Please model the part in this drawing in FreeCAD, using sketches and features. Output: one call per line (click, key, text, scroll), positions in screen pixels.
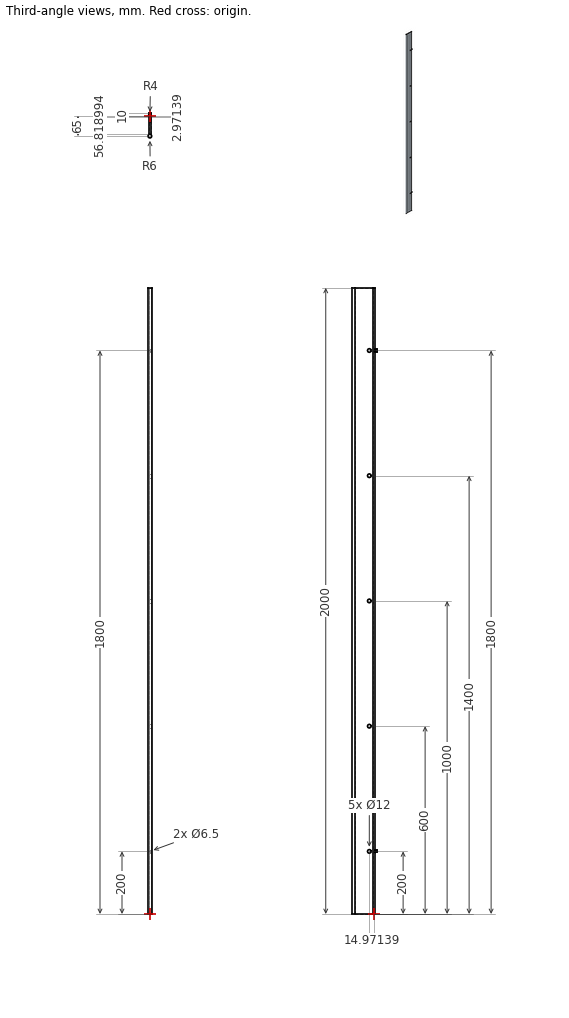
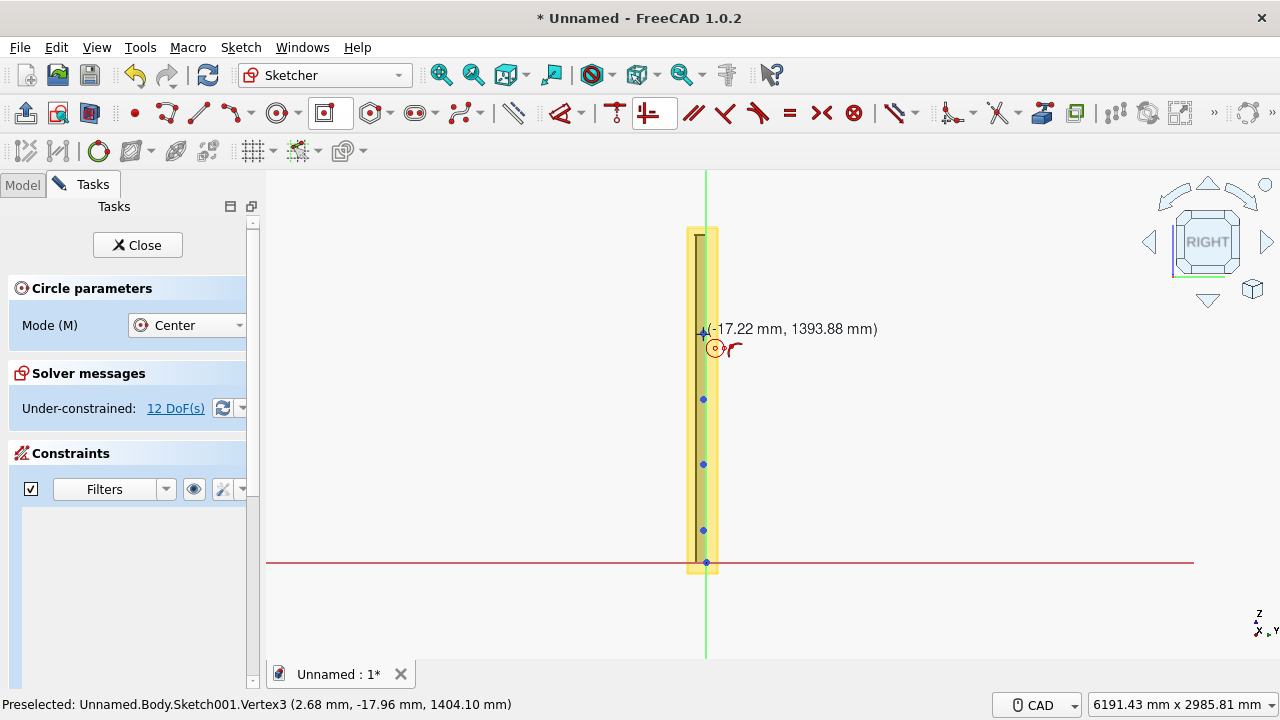
scroll(704, 268, up, 16)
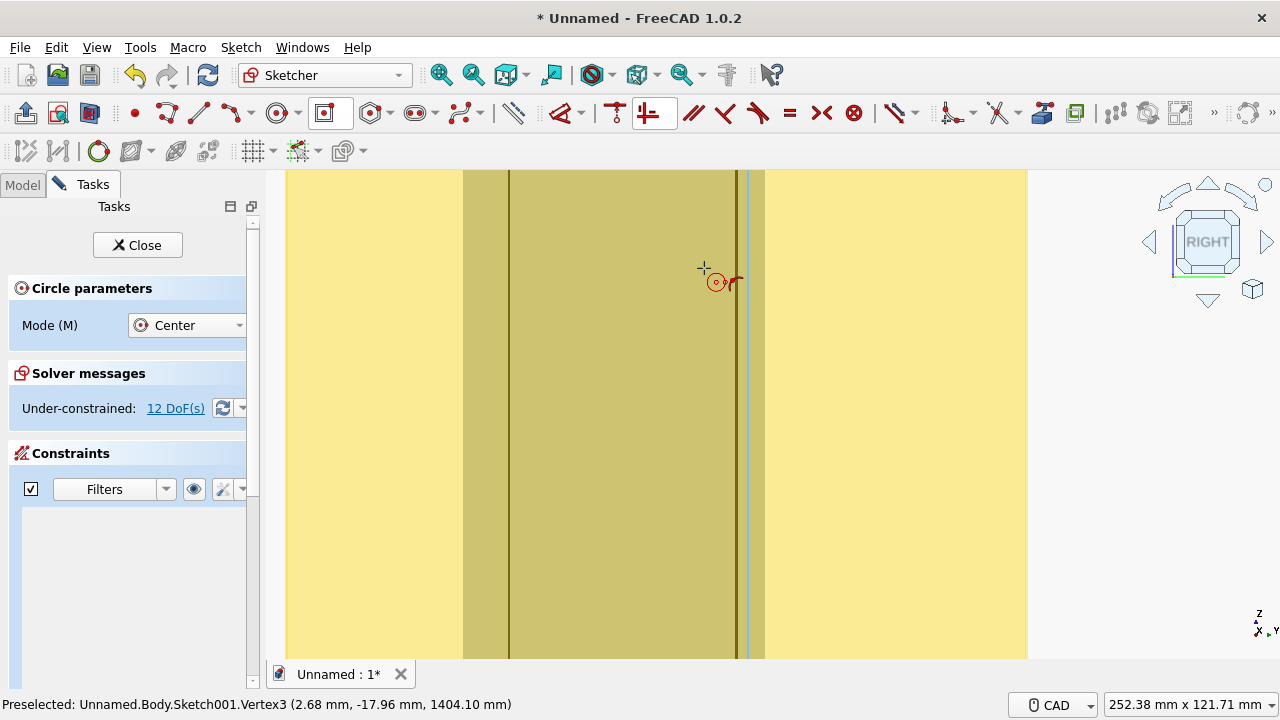
scroll(704, 234, down, 15)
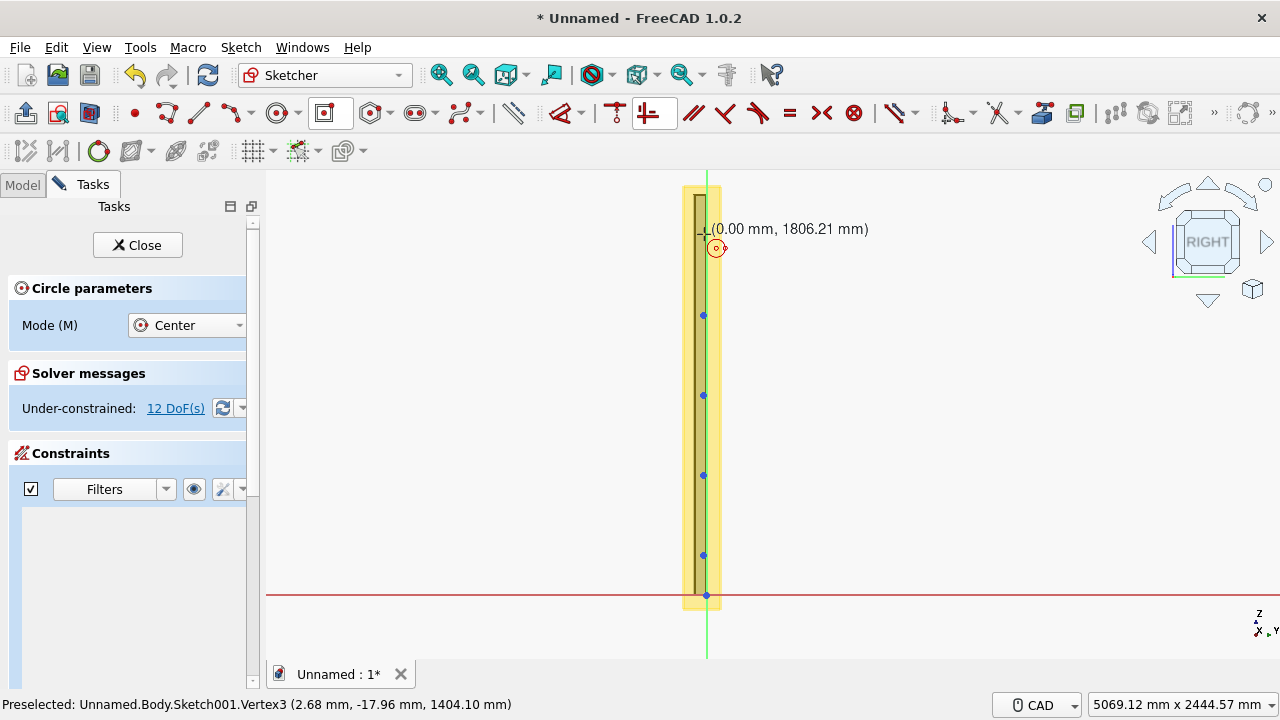
scroll(704, 235, up, 9)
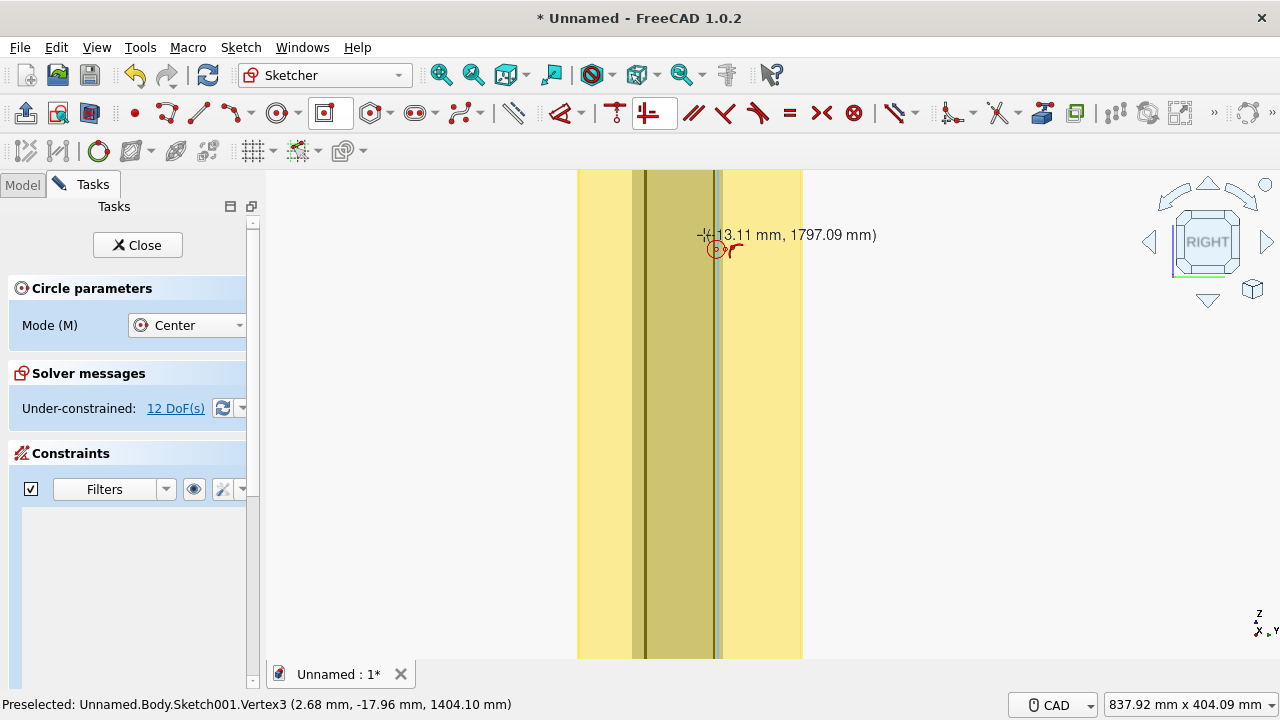
click(700, 237)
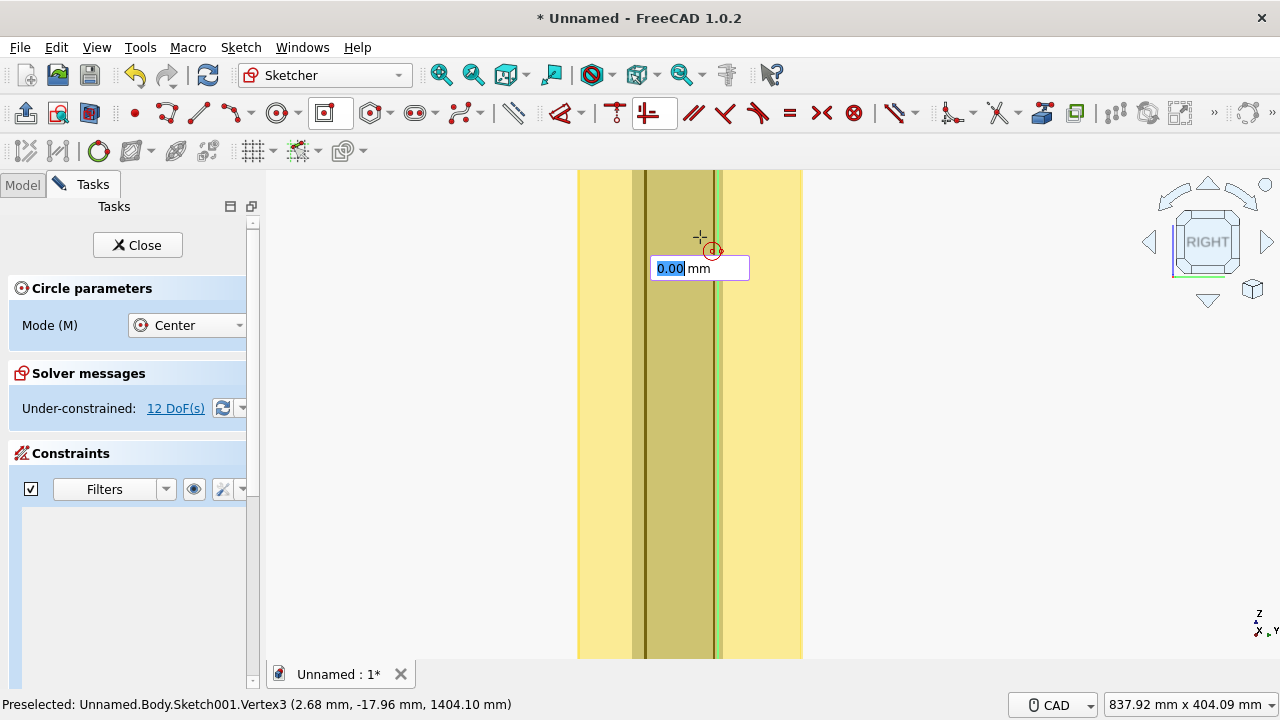
scroll(694, 232, up, 4)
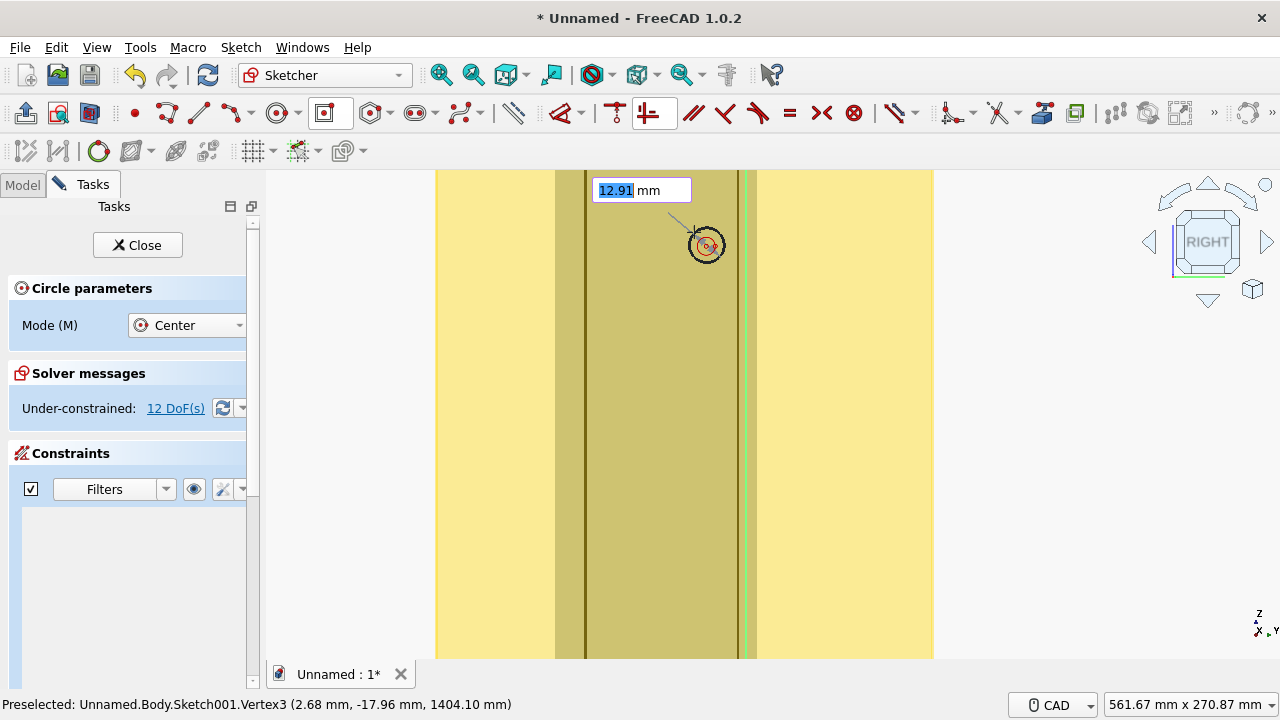
click(694, 231)
key(Escape)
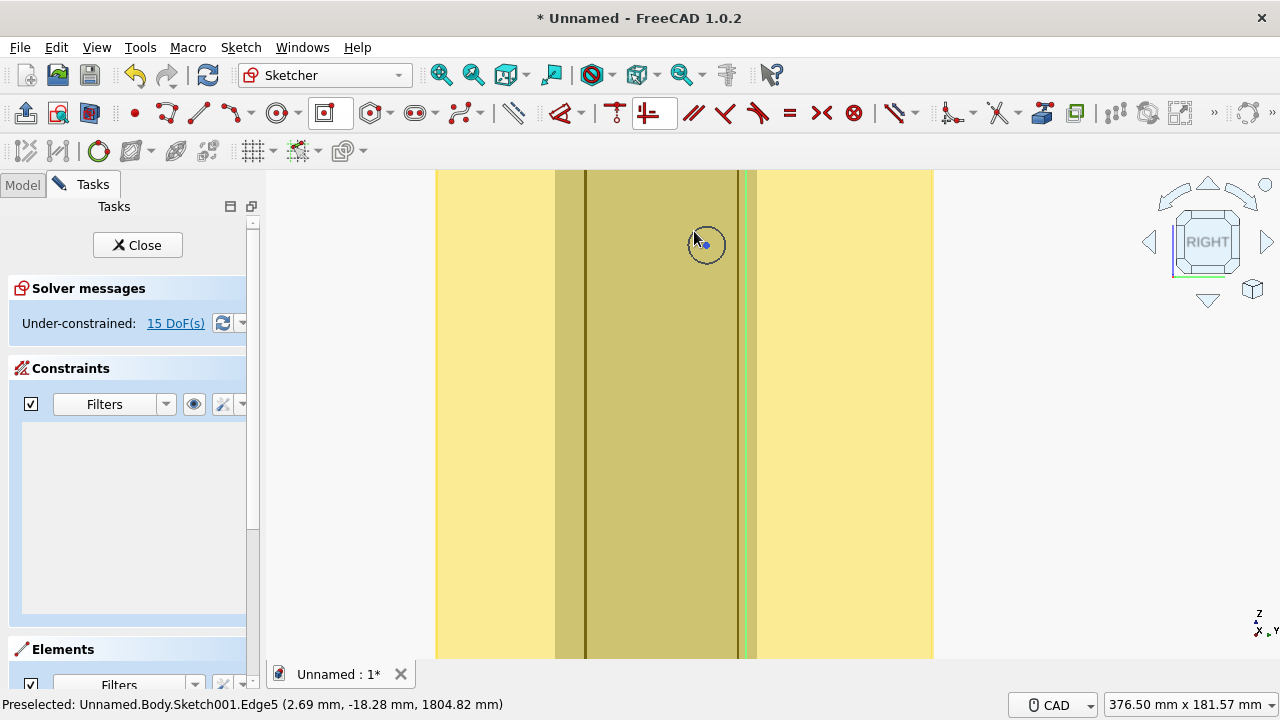
scroll(704, 269, down, 14)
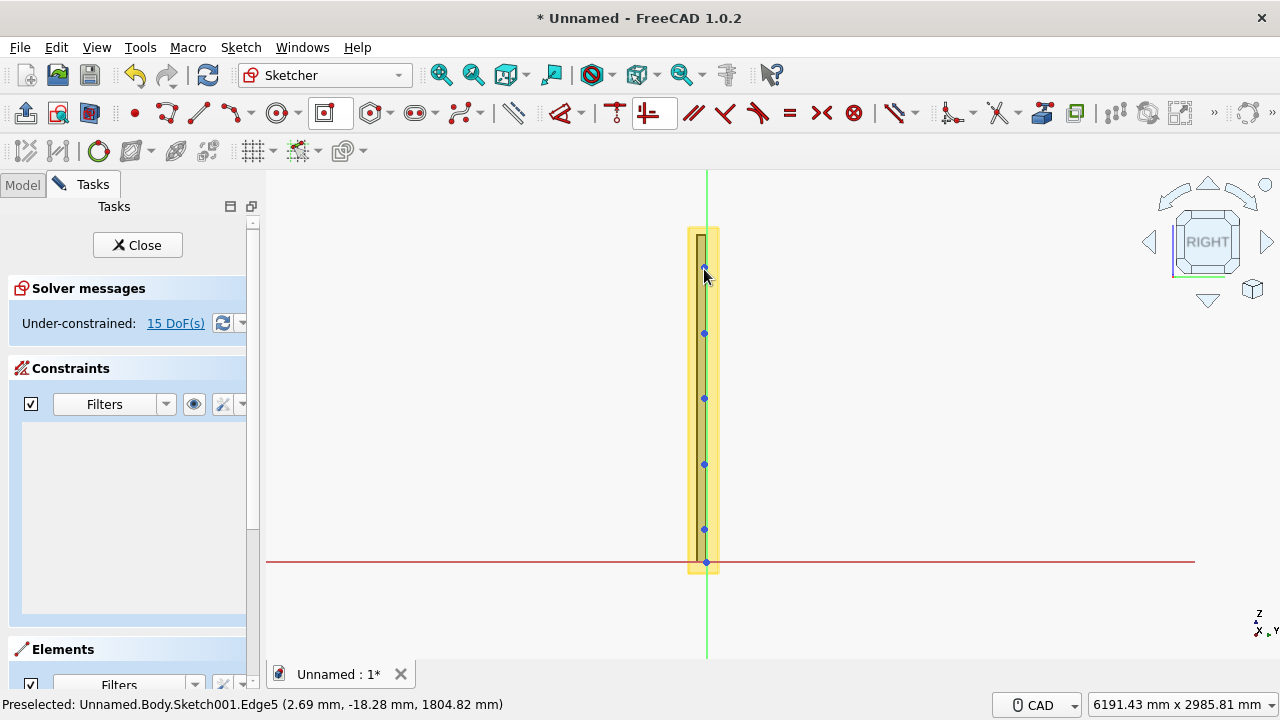
scroll(705, 529, up, 13)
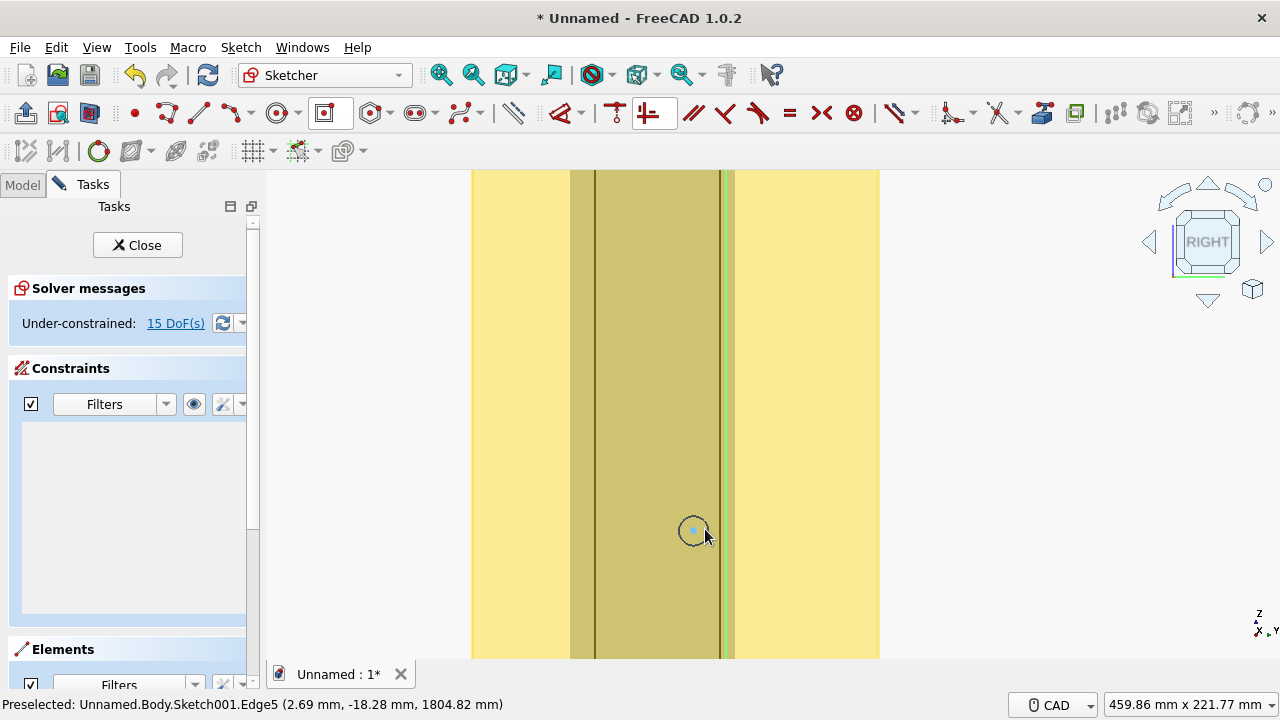
click(704, 521)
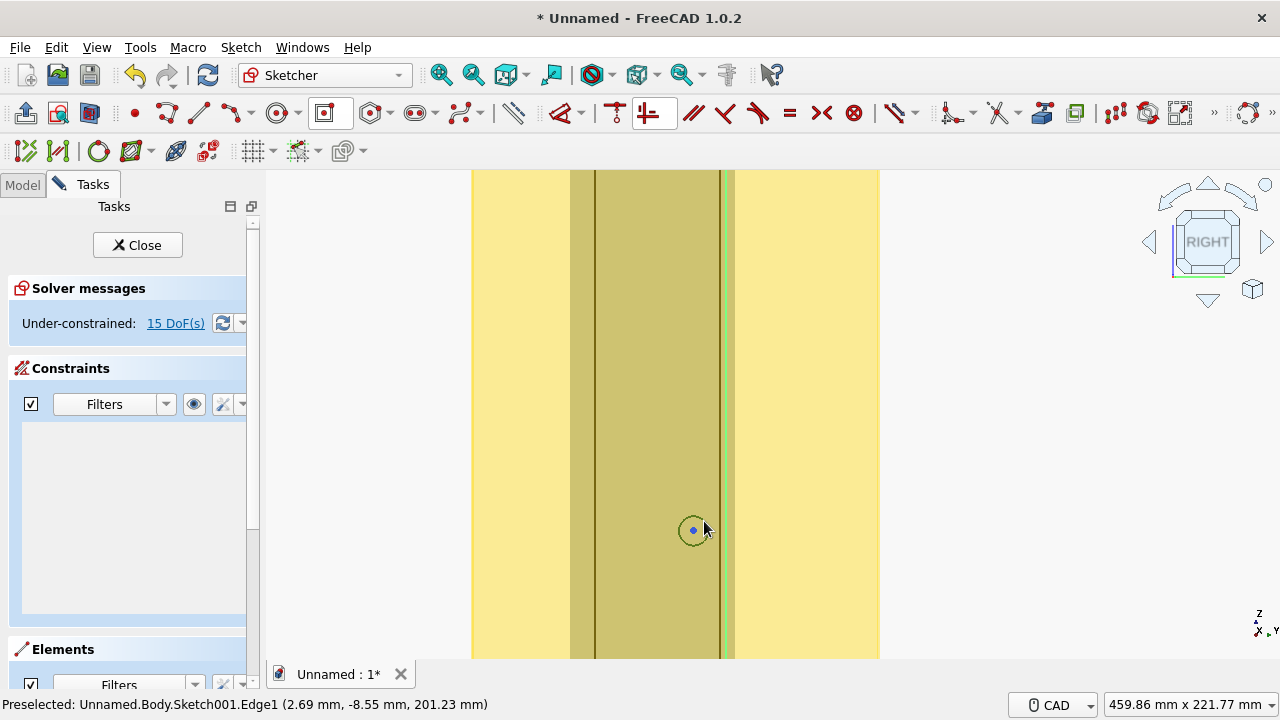
scroll(705, 530, down, 13)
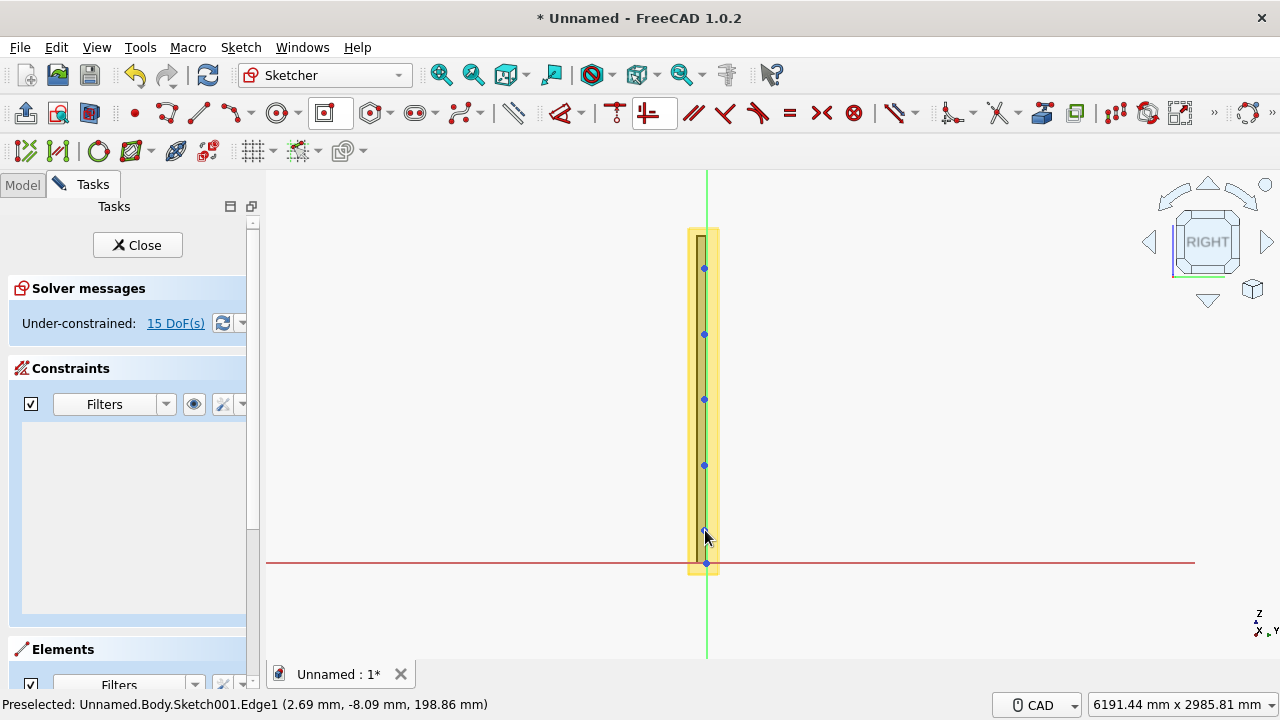
scroll(705, 464, up, 13)